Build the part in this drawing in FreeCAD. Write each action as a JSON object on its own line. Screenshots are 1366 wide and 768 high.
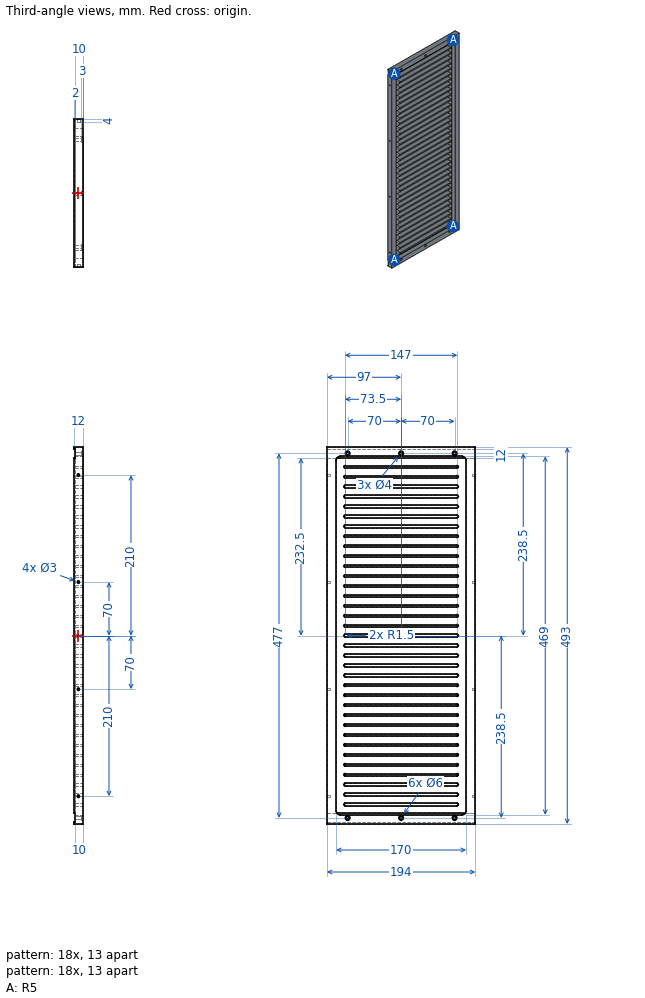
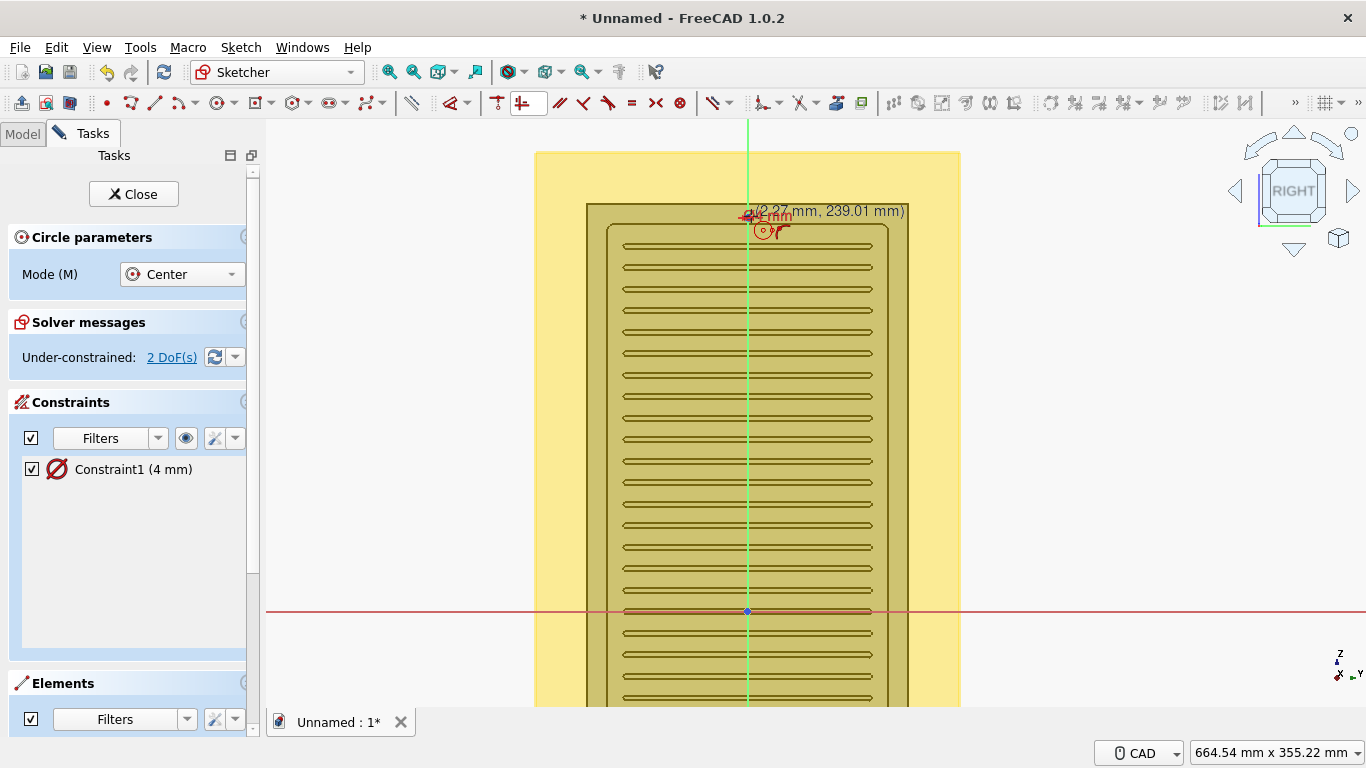
{"action": "scroll", "coordinate": [863, 217], "scroll_direction": "up", "scroll_amount": 10}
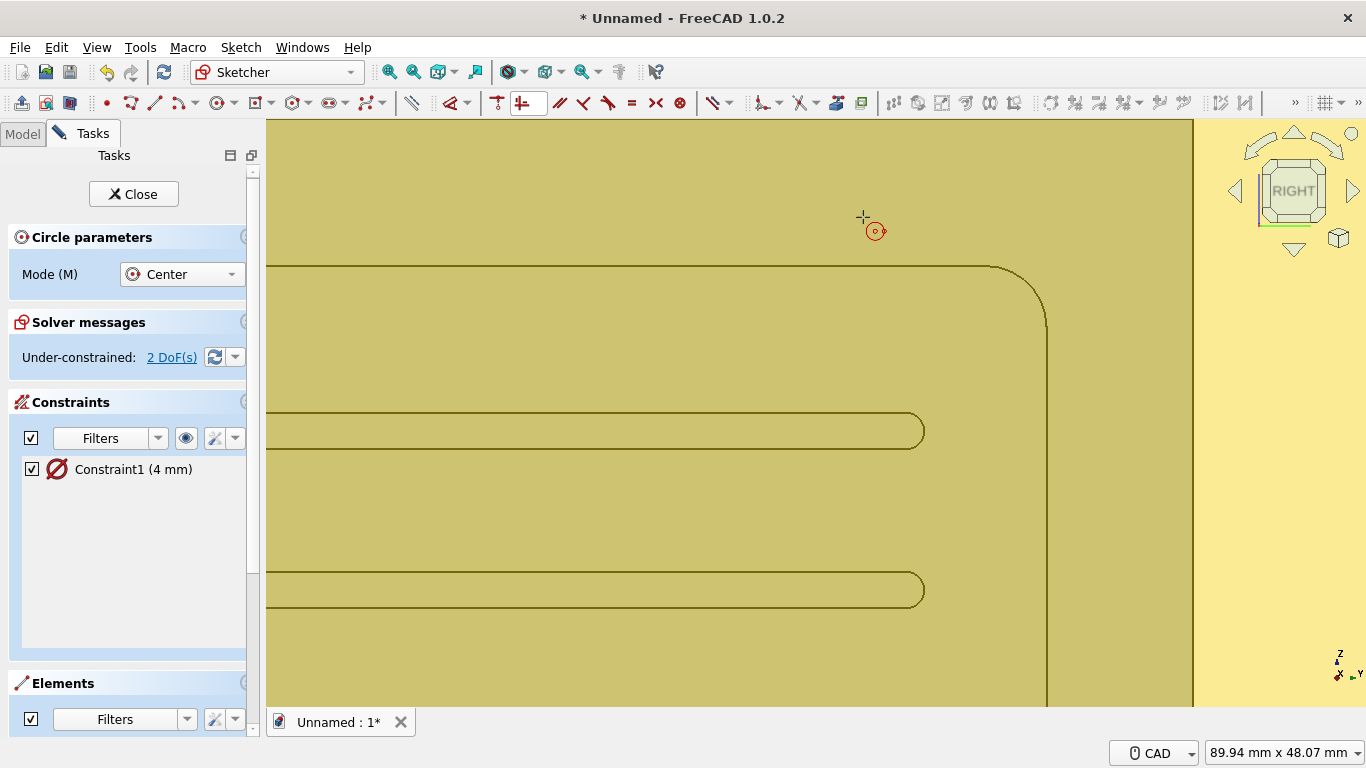
{"action": "scroll", "coordinate": [863, 217], "scroll_direction": "down", "scroll_amount": 10}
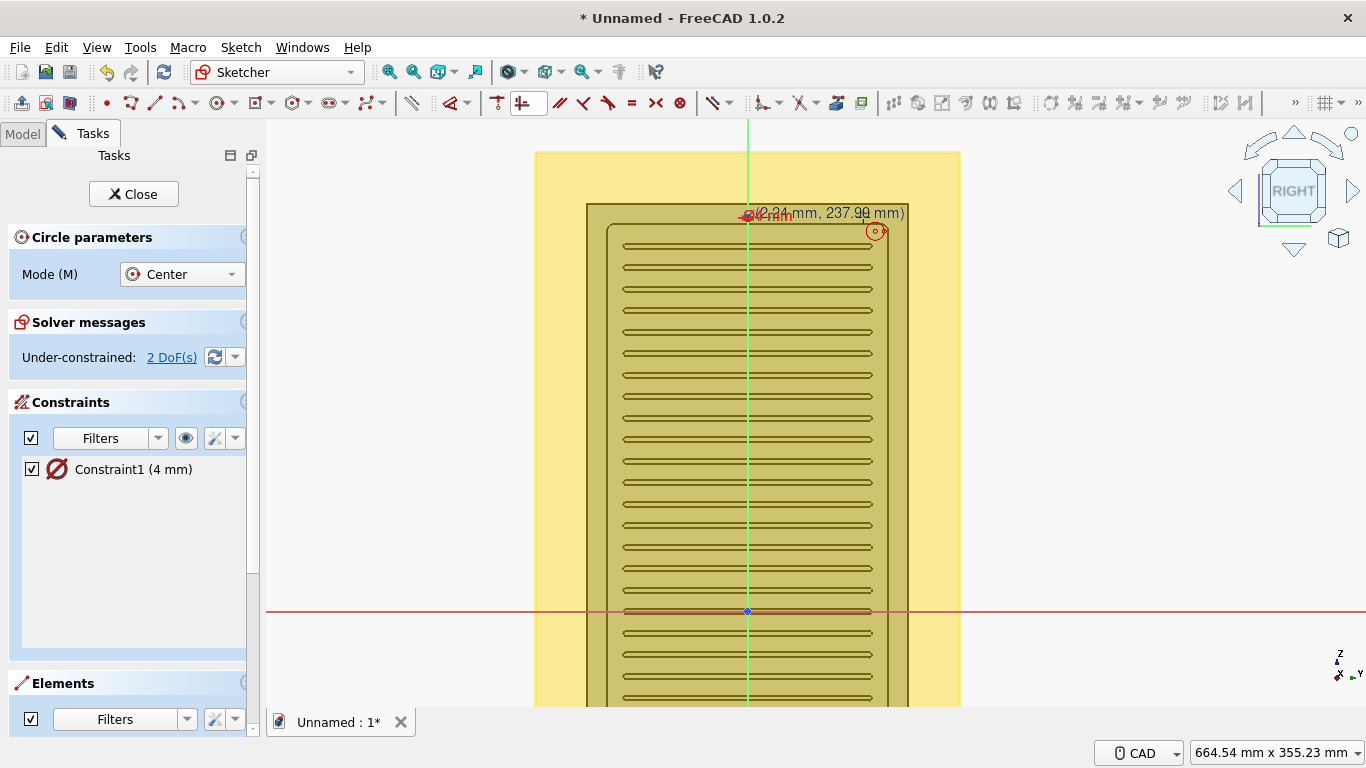
{"action": "left_click", "coordinate": [863, 217]}
{"action": "mouse_move", "coordinate": [866, 215]}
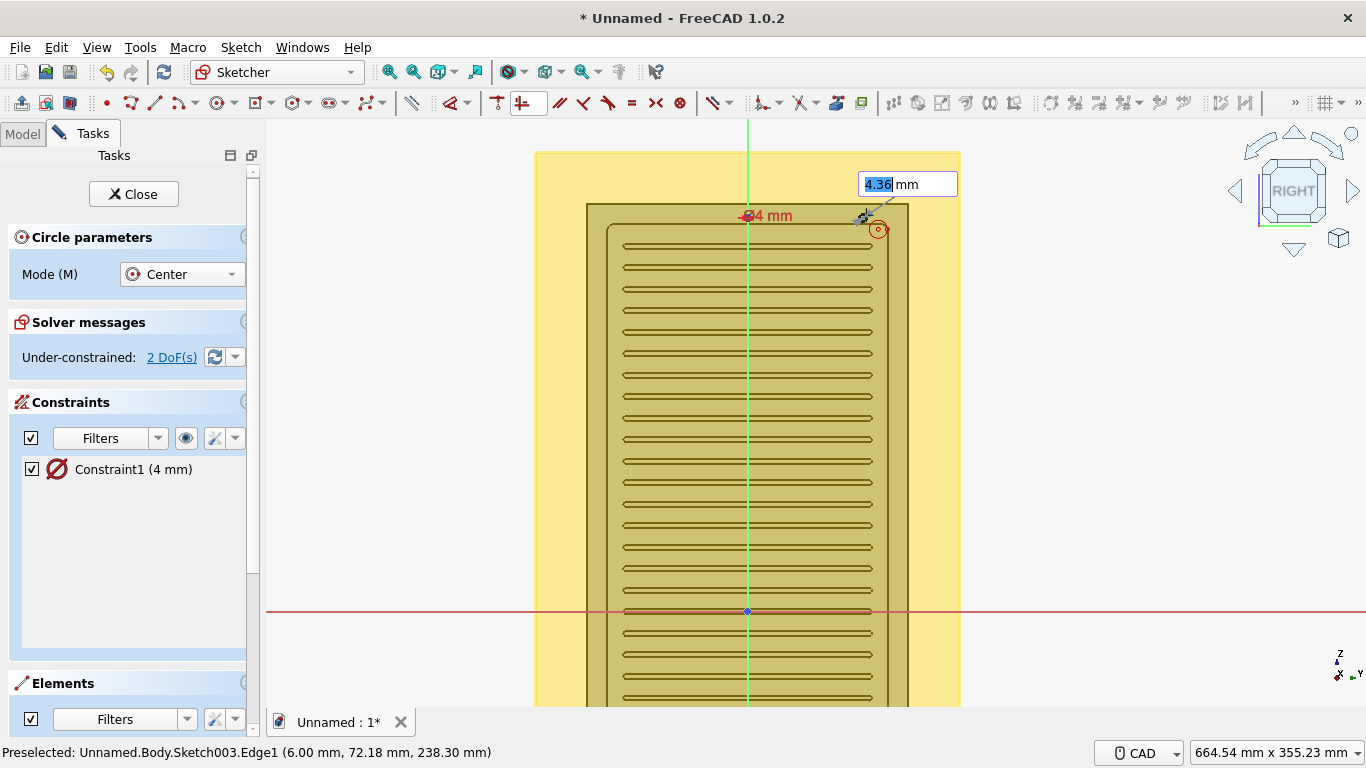
{"action": "type", "text": "4"}
{"action": "key", "text": "Return"}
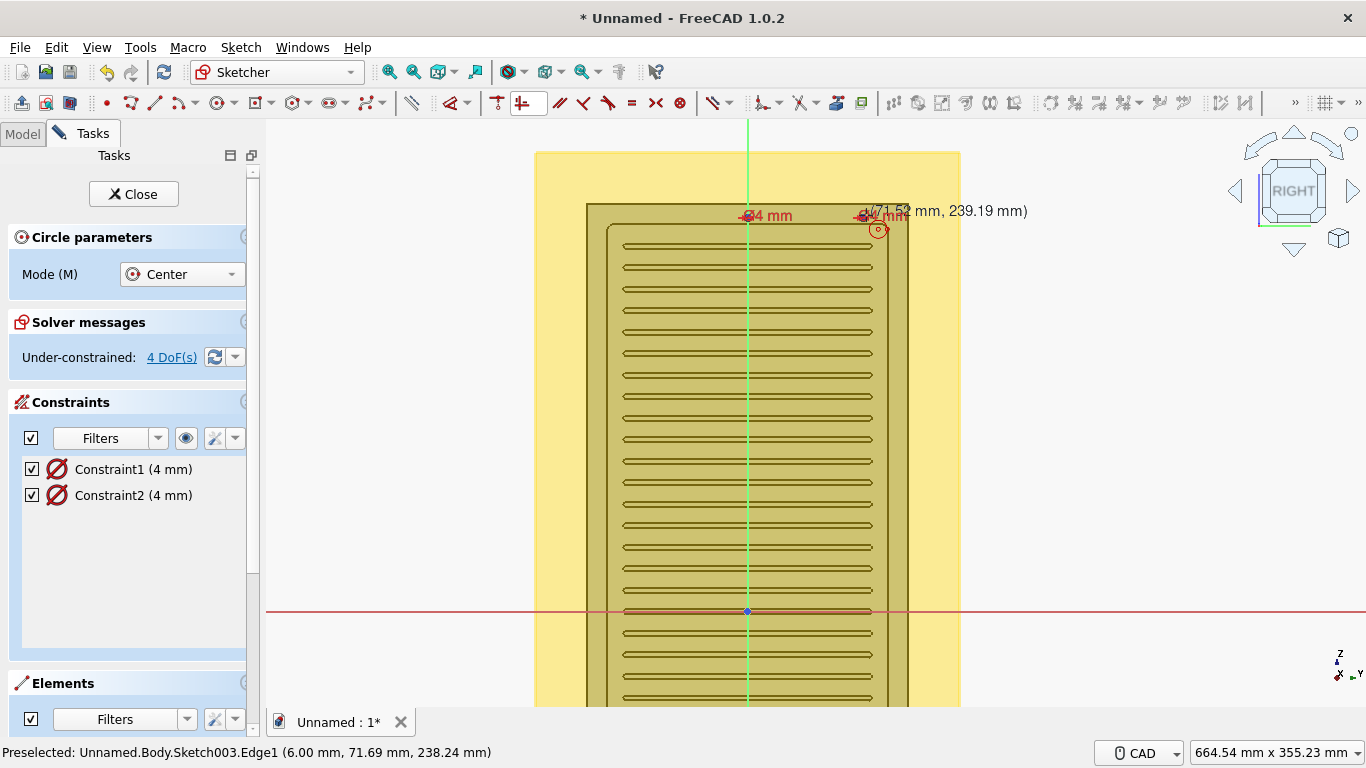
{"action": "scroll", "coordinate": [632, 217], "scroll_direction": "up", "scroll_amount": 10}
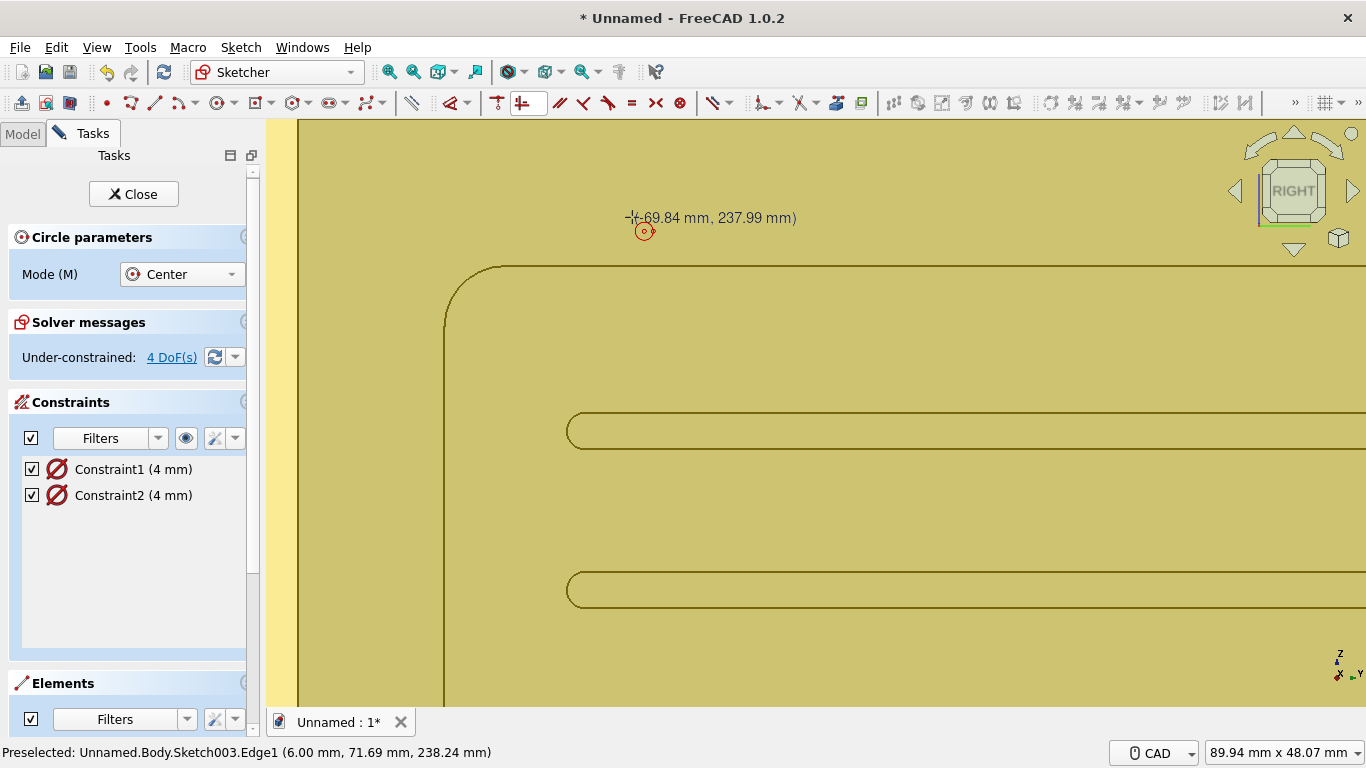
{"action": "scroll", "coordinate": [632, 217], "scroll_direction": "down", "scroll_amount": 10}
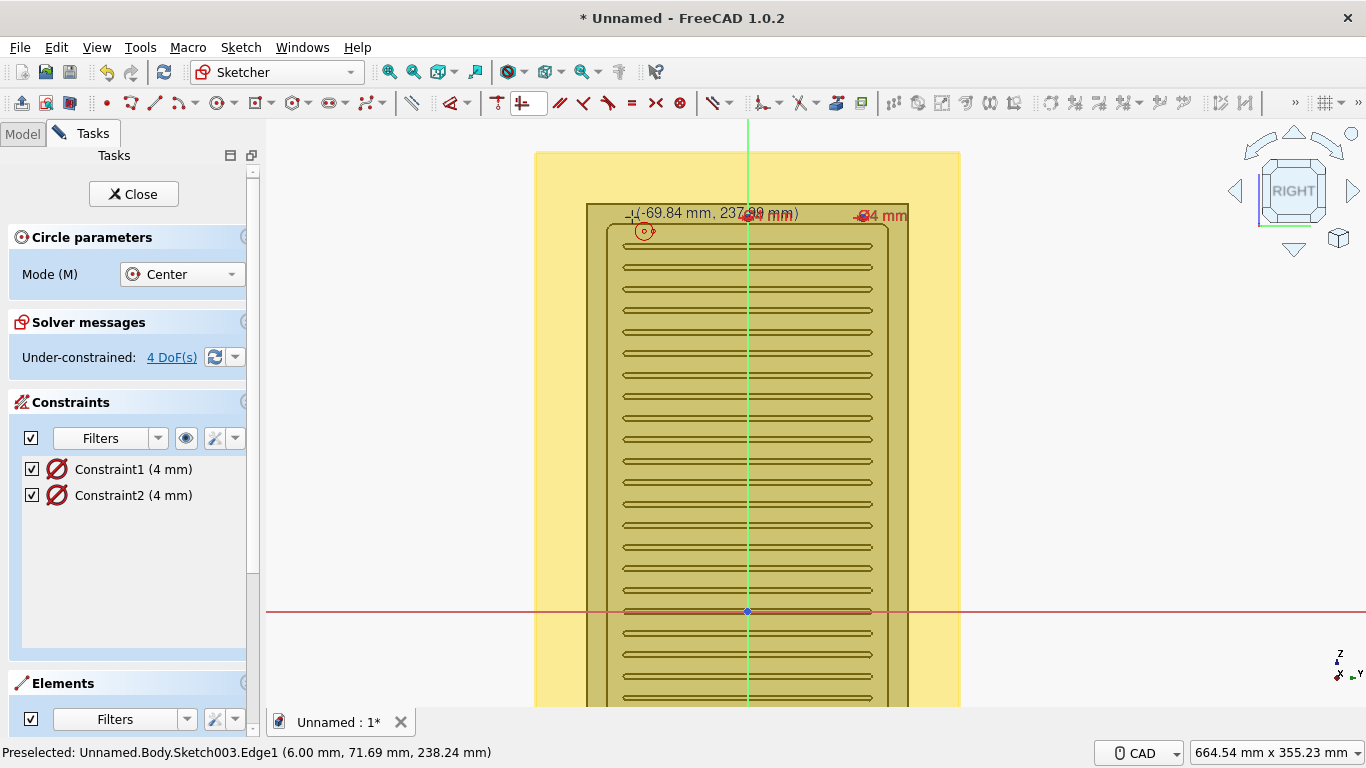
{"action": "left_click", "coordinate": [632, 217]}
{"action": "mouse_move", "coordinate": [634, 215]}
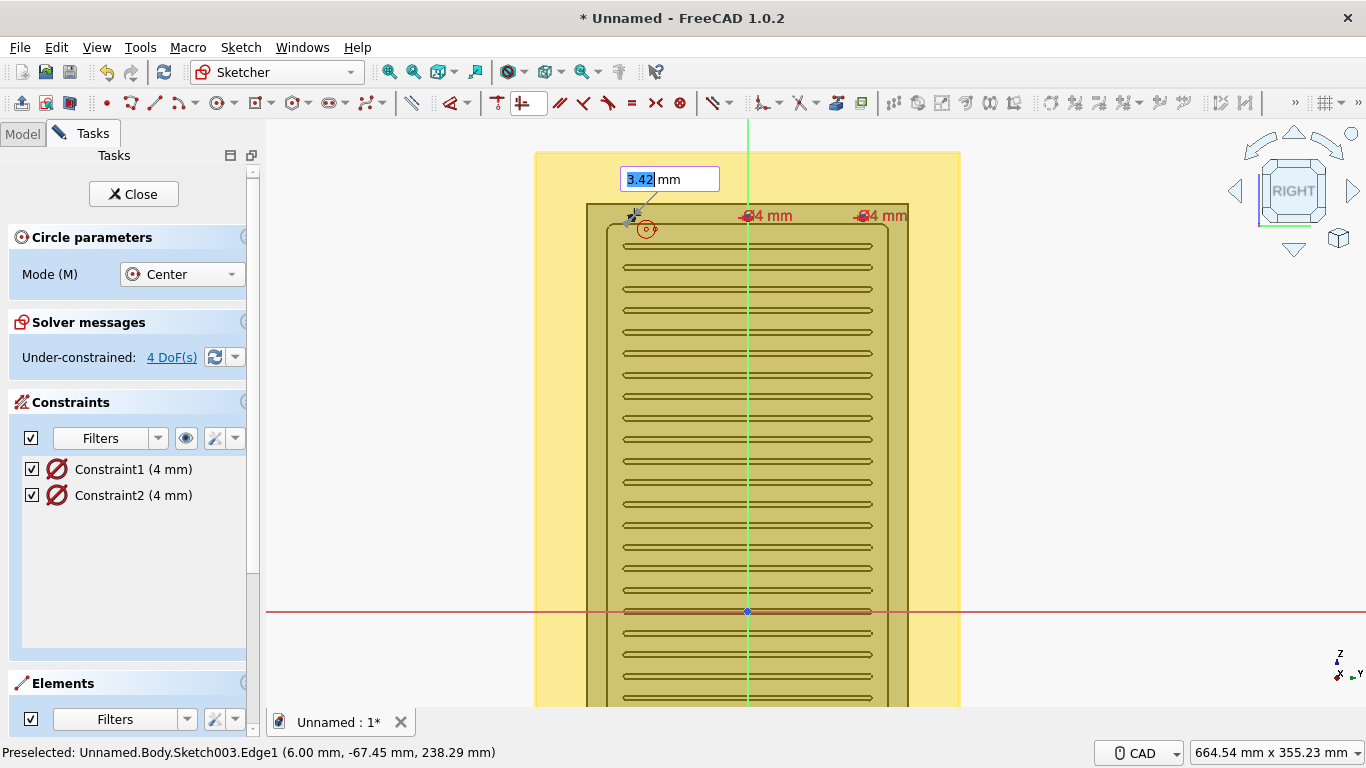
{"action": "type", "text": "4"}
{"action": "key", "text": "Return"}
{"action": "key", "text": "Escape"}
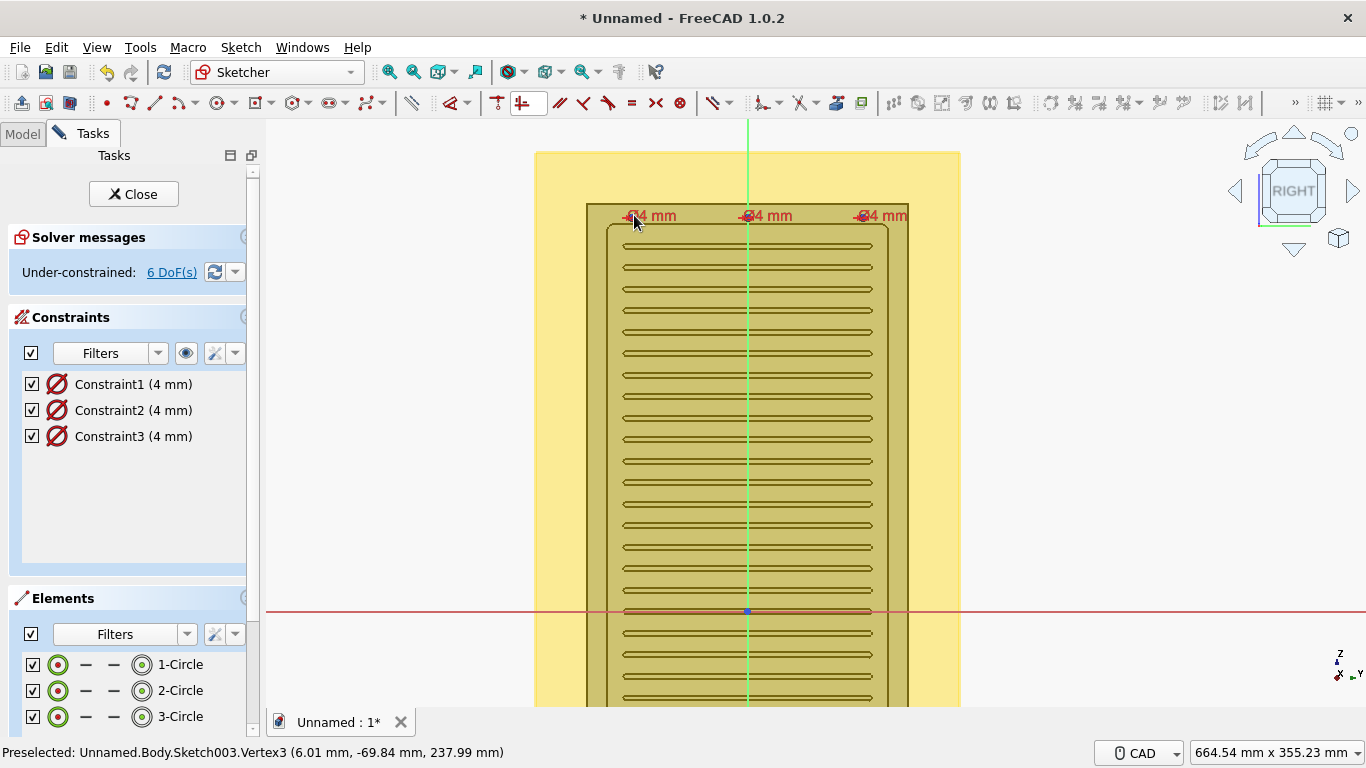
{"action": "left_click", "coordinate": [748, 218]}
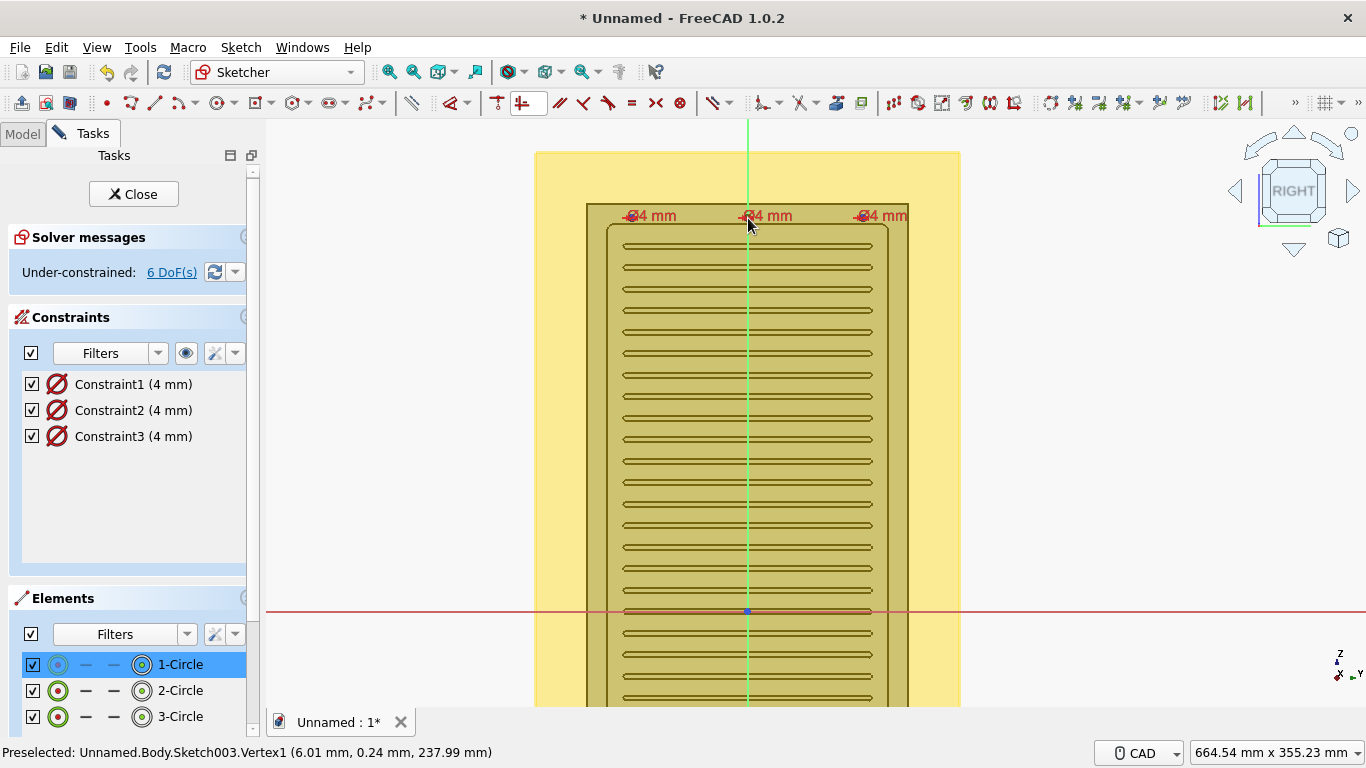
{"action": "left_click", "coordinate": [748, 565]}